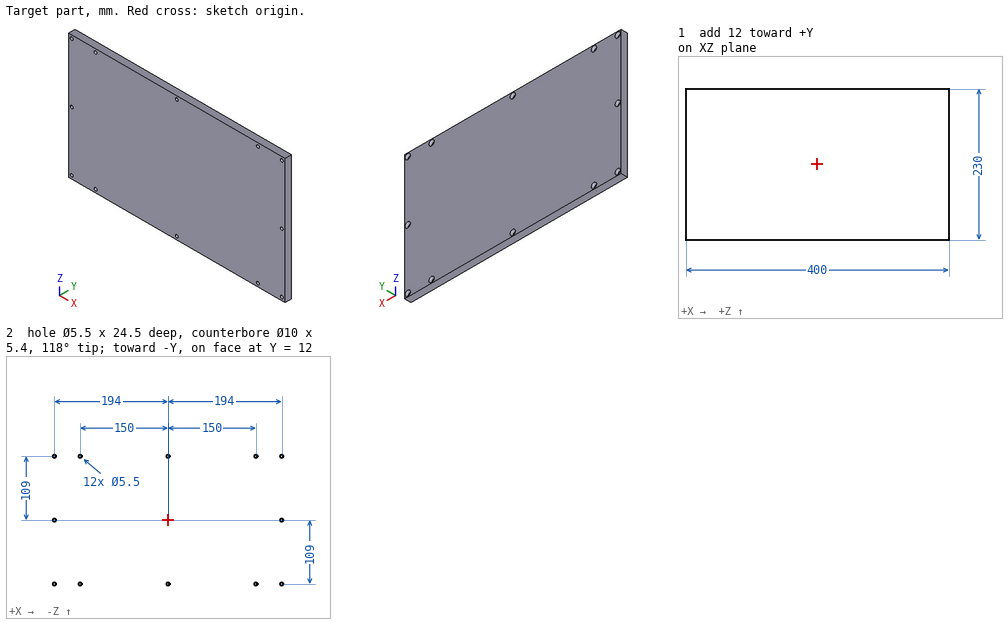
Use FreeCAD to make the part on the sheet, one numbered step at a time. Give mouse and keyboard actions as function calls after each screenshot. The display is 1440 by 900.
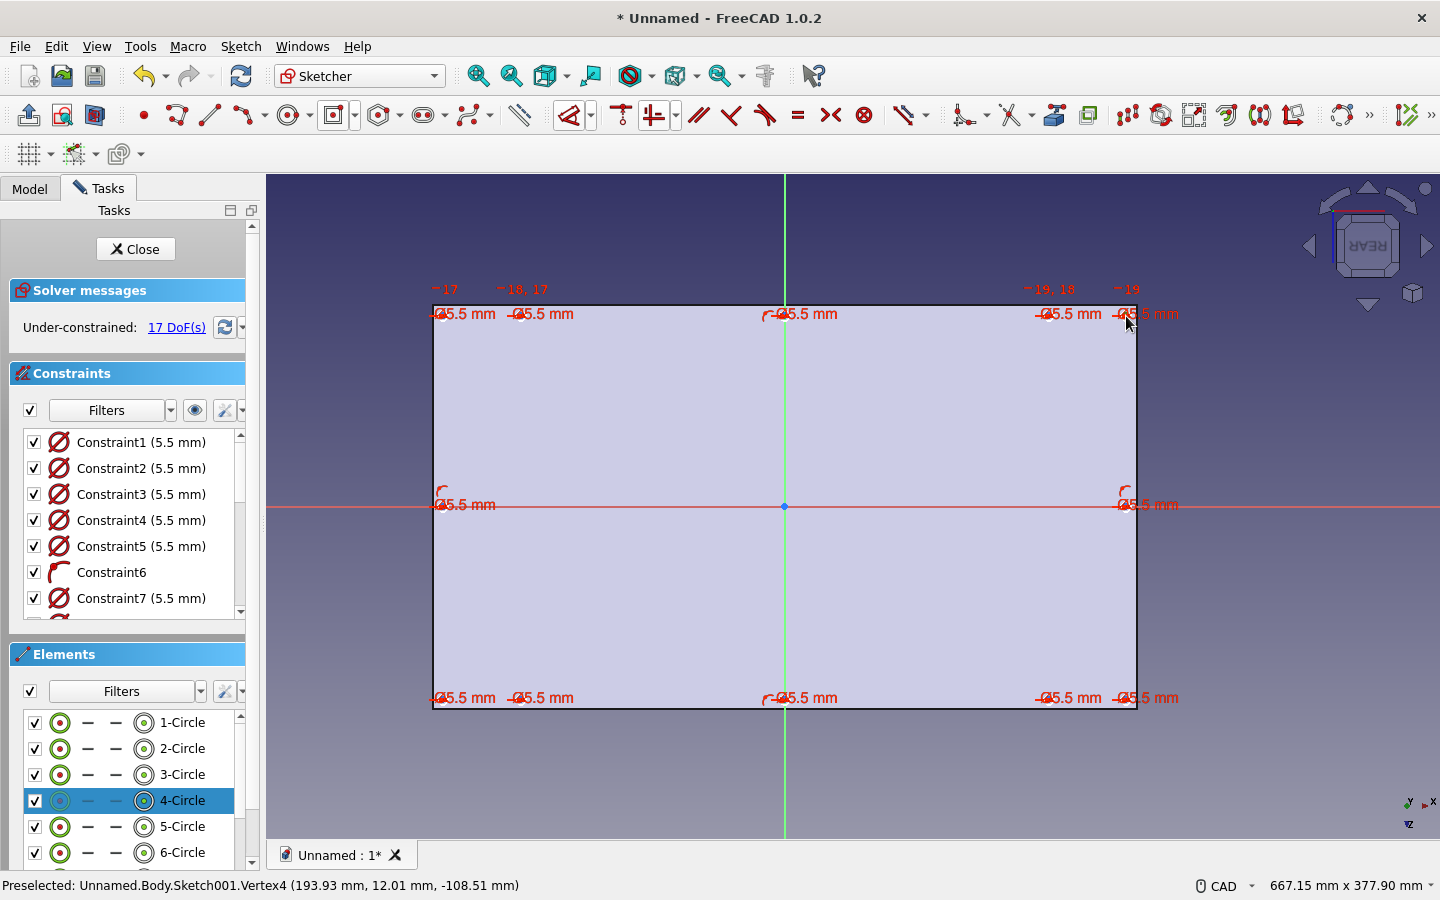
click(1126, 507)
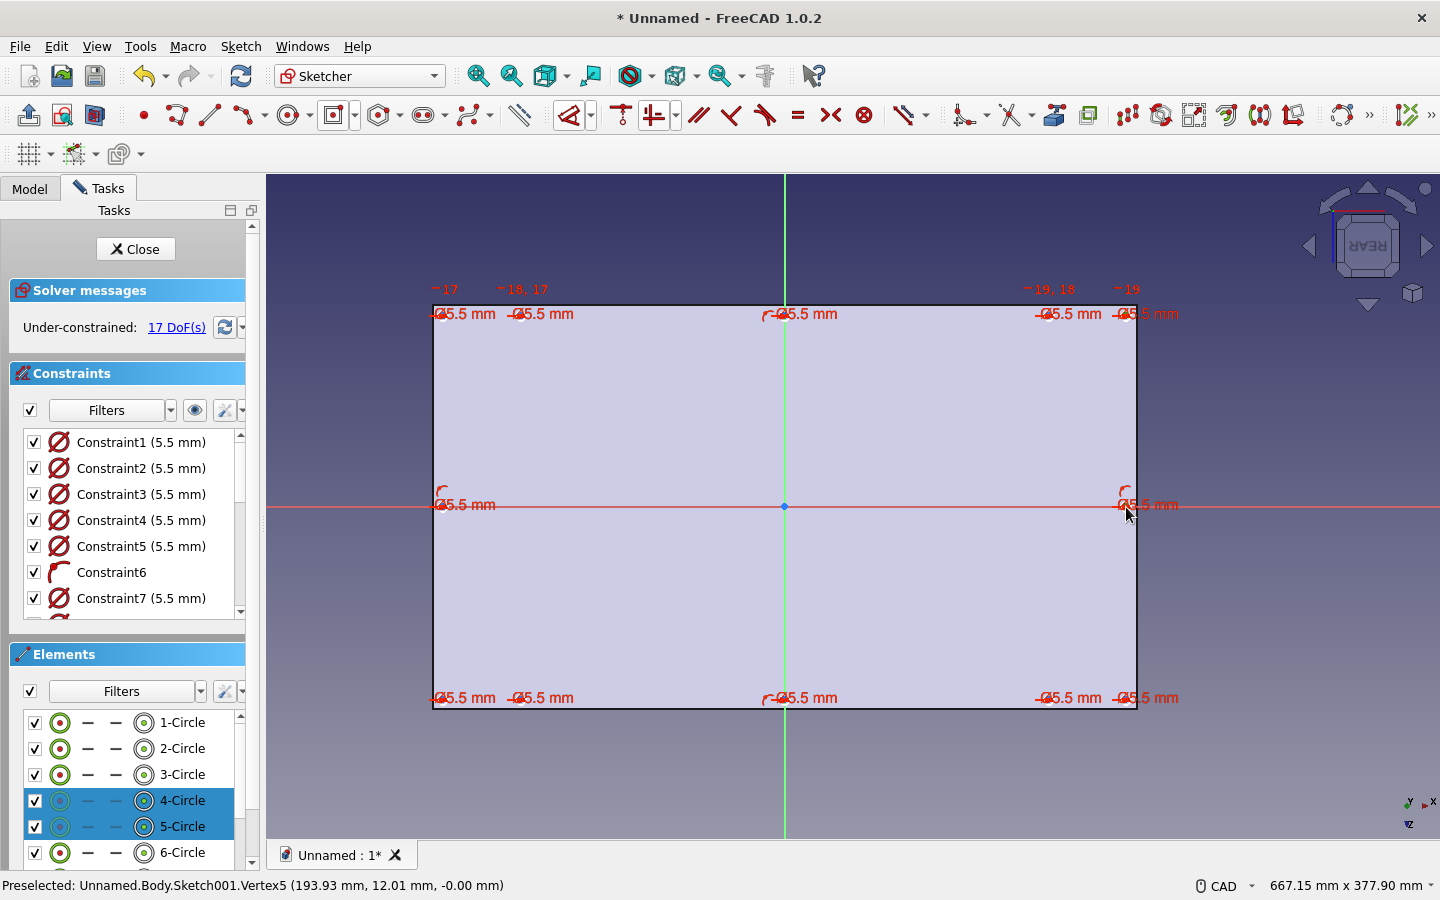
click(676, 116)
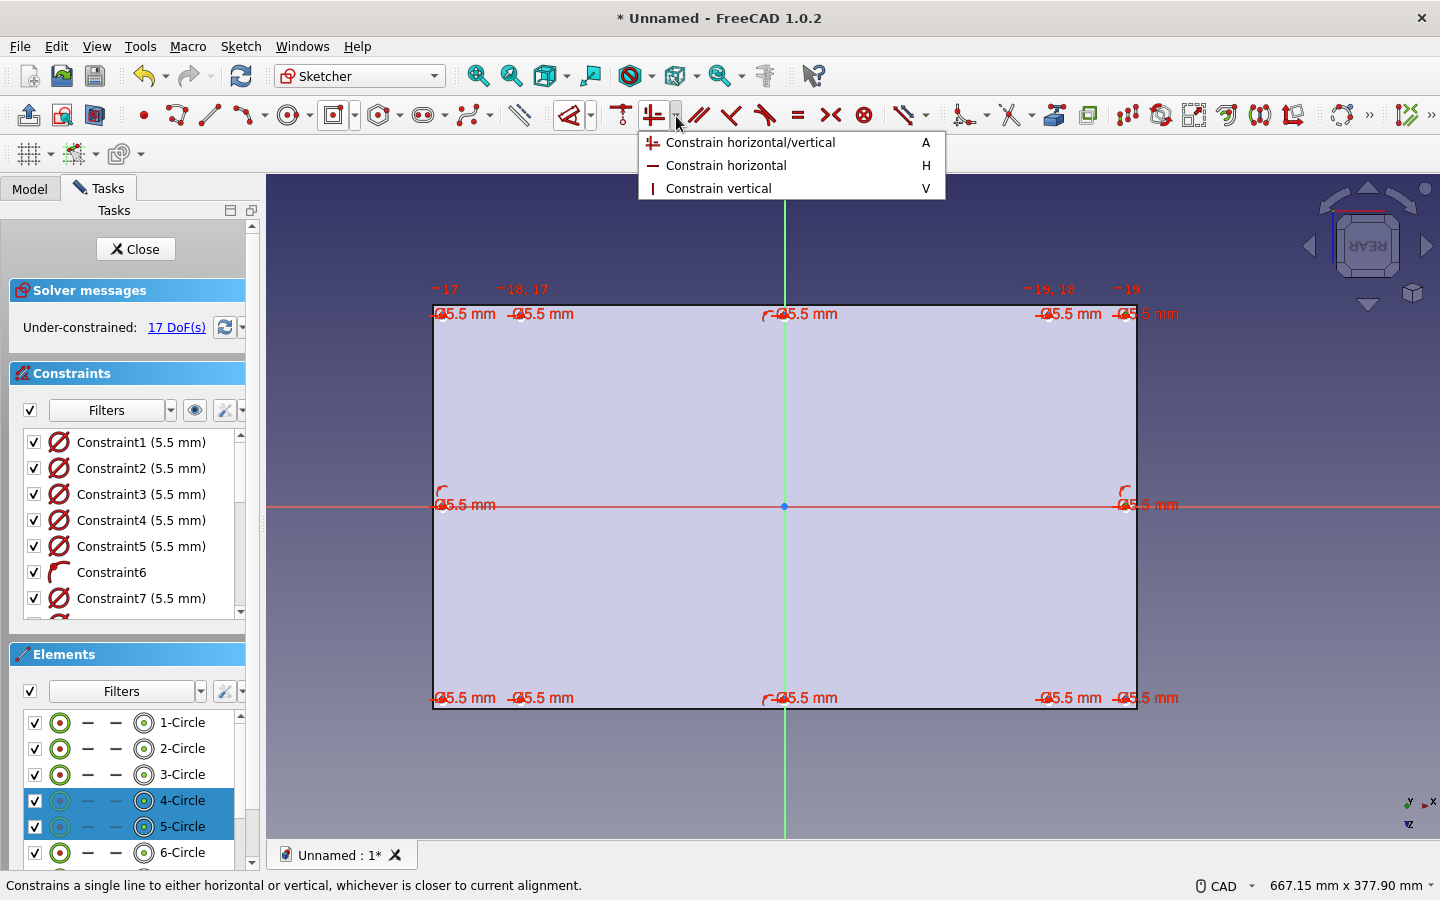
click(792, 188)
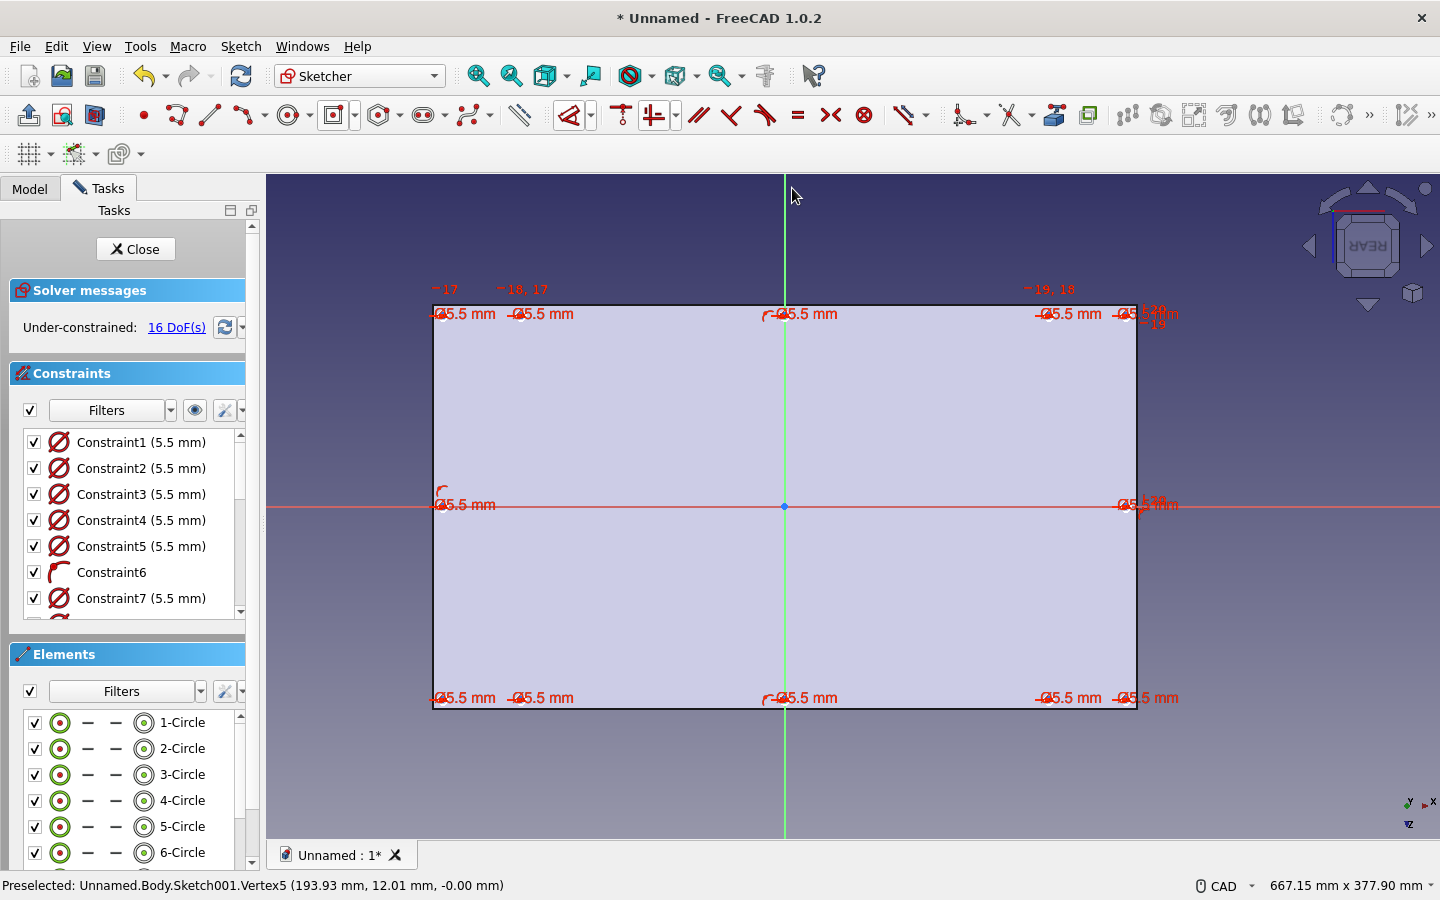
click(1126, 507)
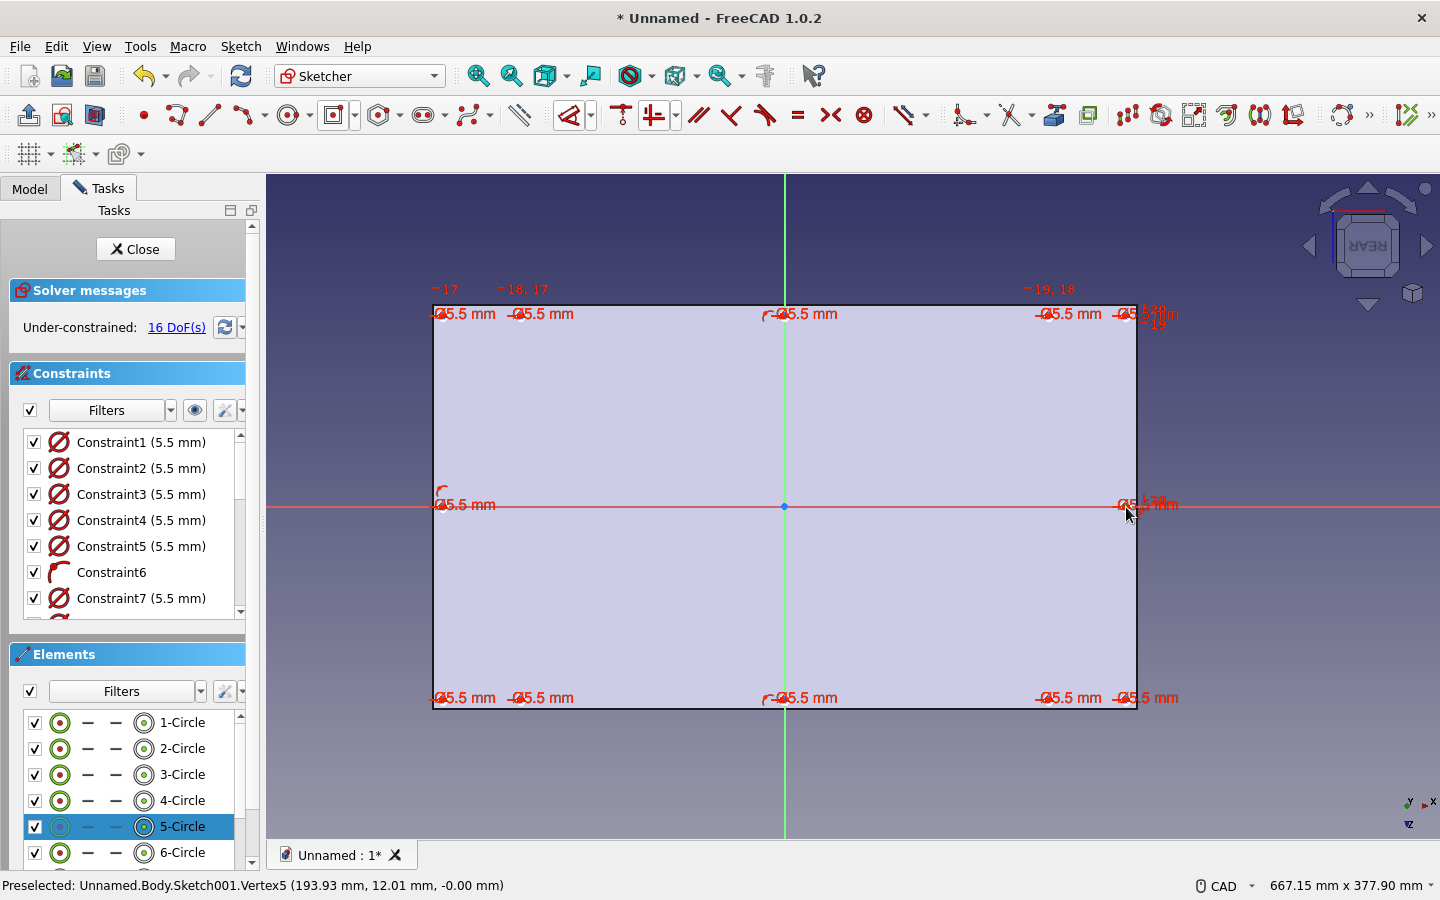
click(1126, 700)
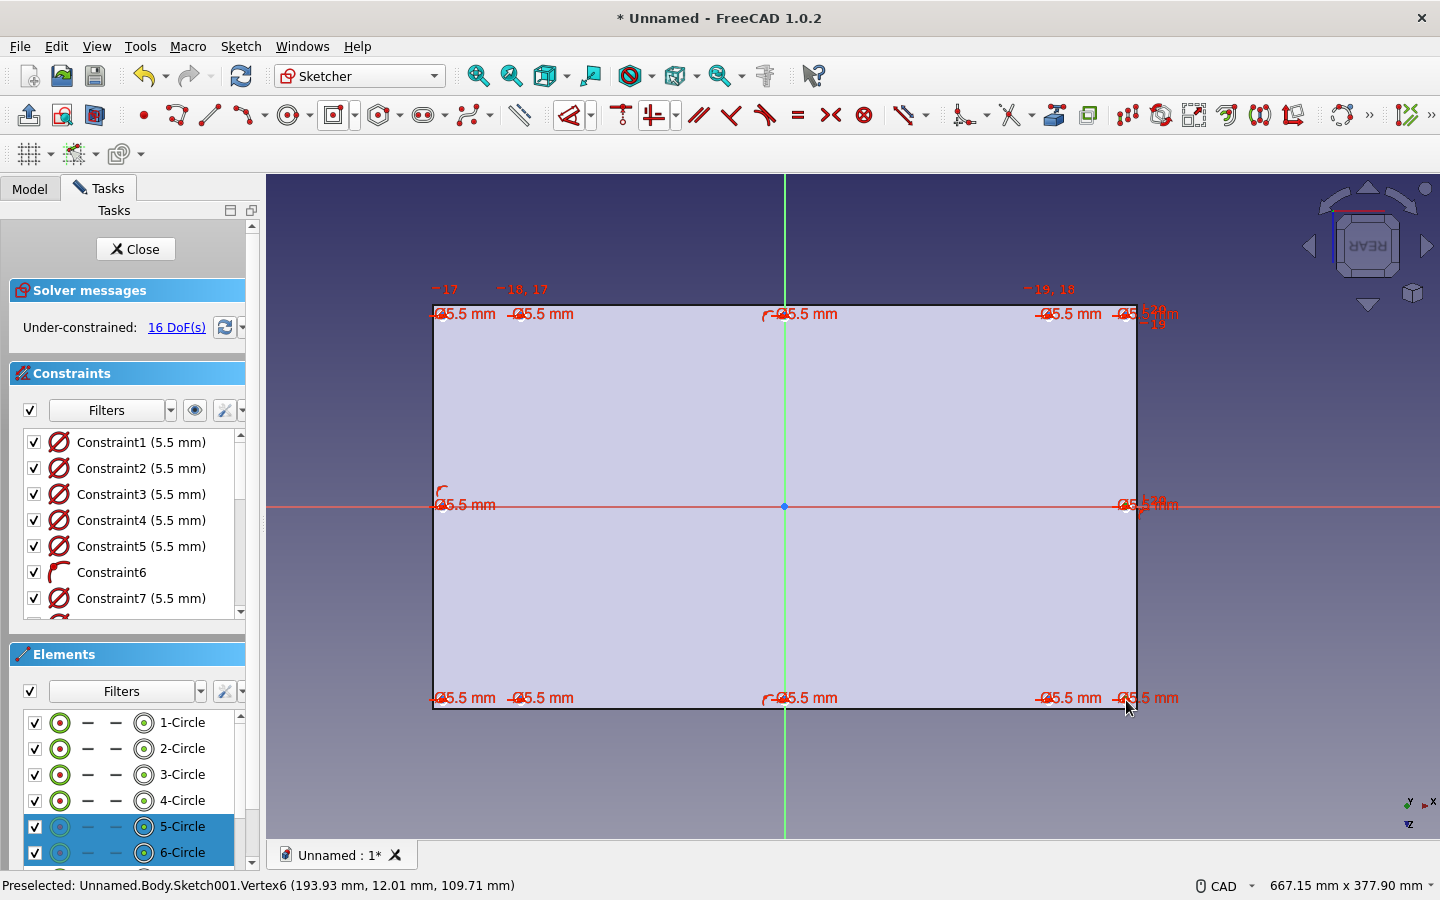
click(676, 116)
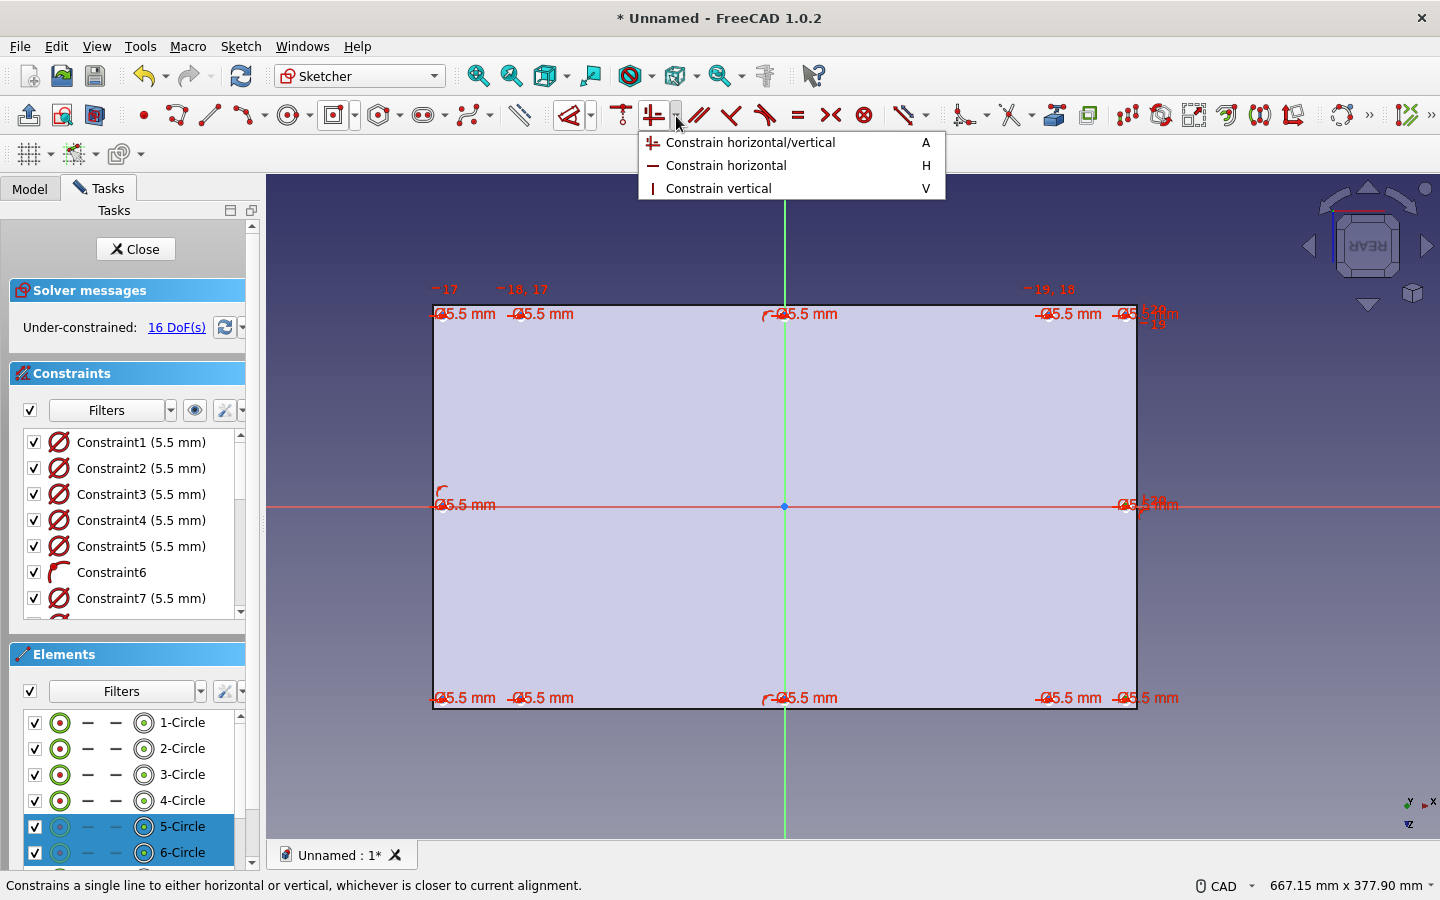
click(792, 188)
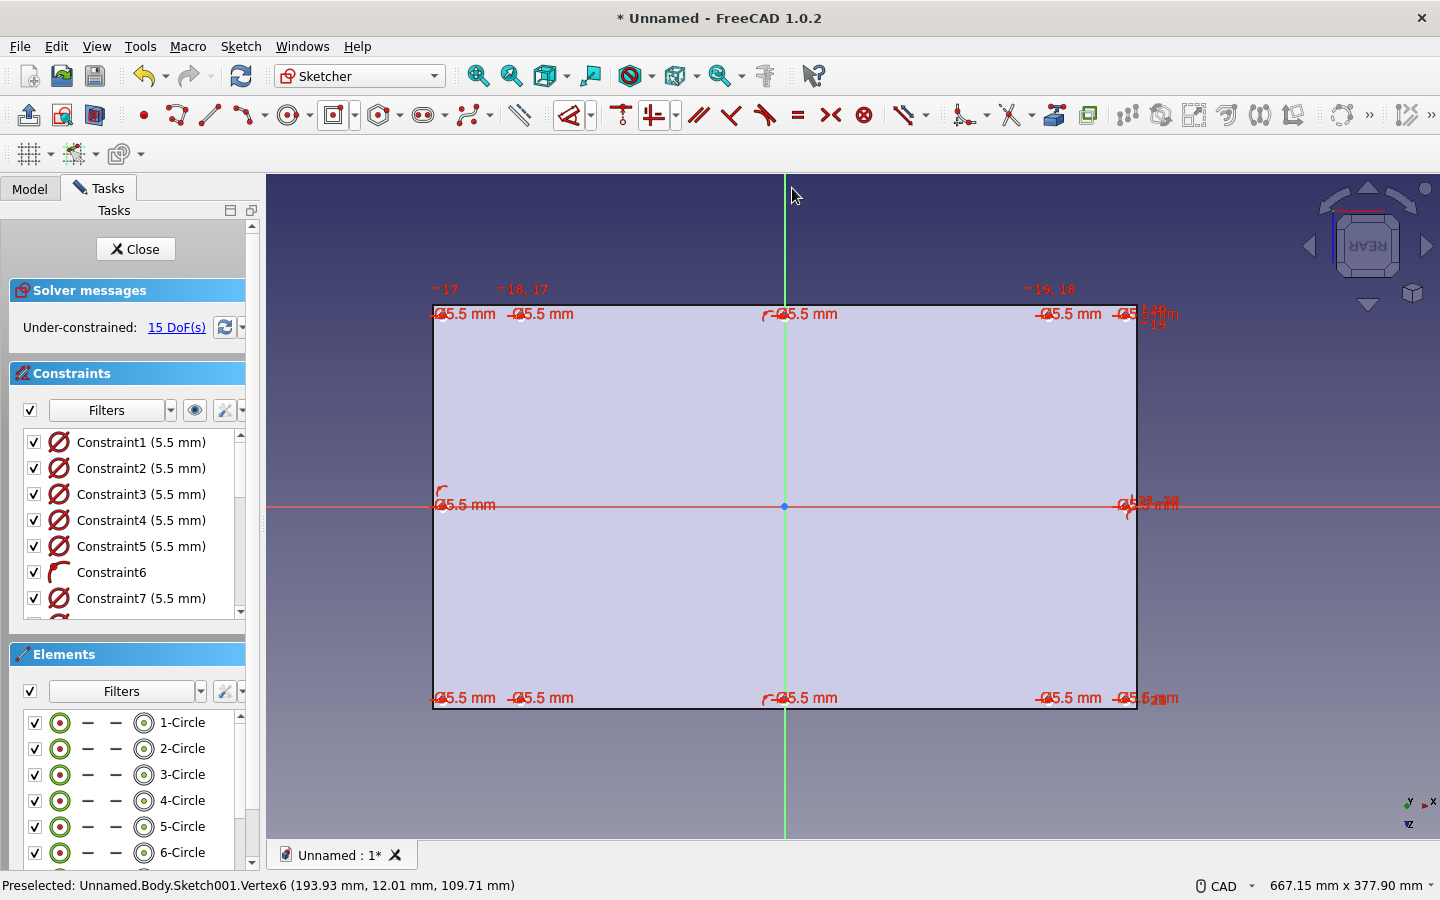
click(1049, 316)